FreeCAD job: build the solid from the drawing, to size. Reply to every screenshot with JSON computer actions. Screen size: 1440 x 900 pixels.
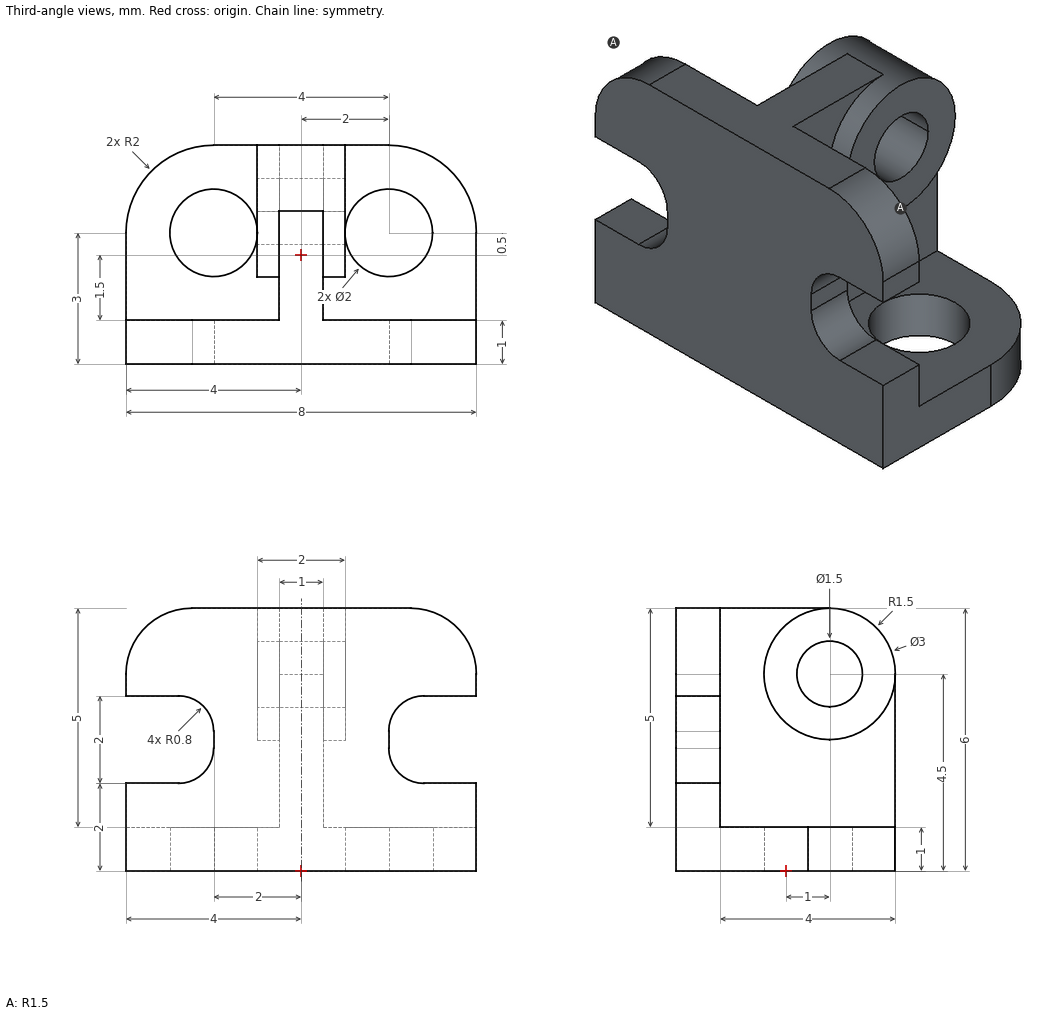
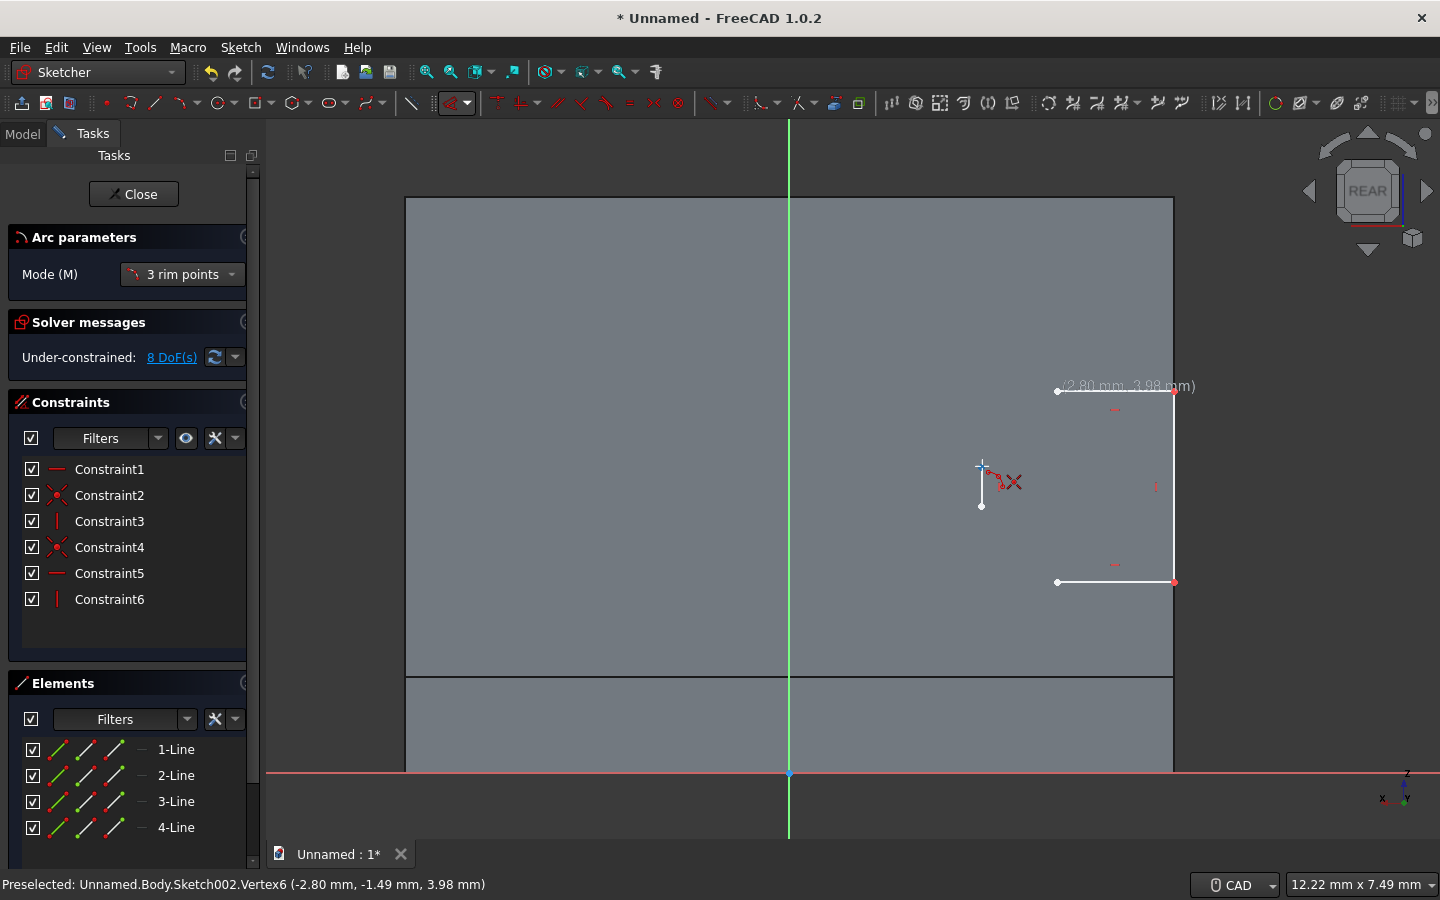
{"action": "left_click", "coordinate": [982, 467]}
{"action": "left_click", "coordinate": [1004, 412]}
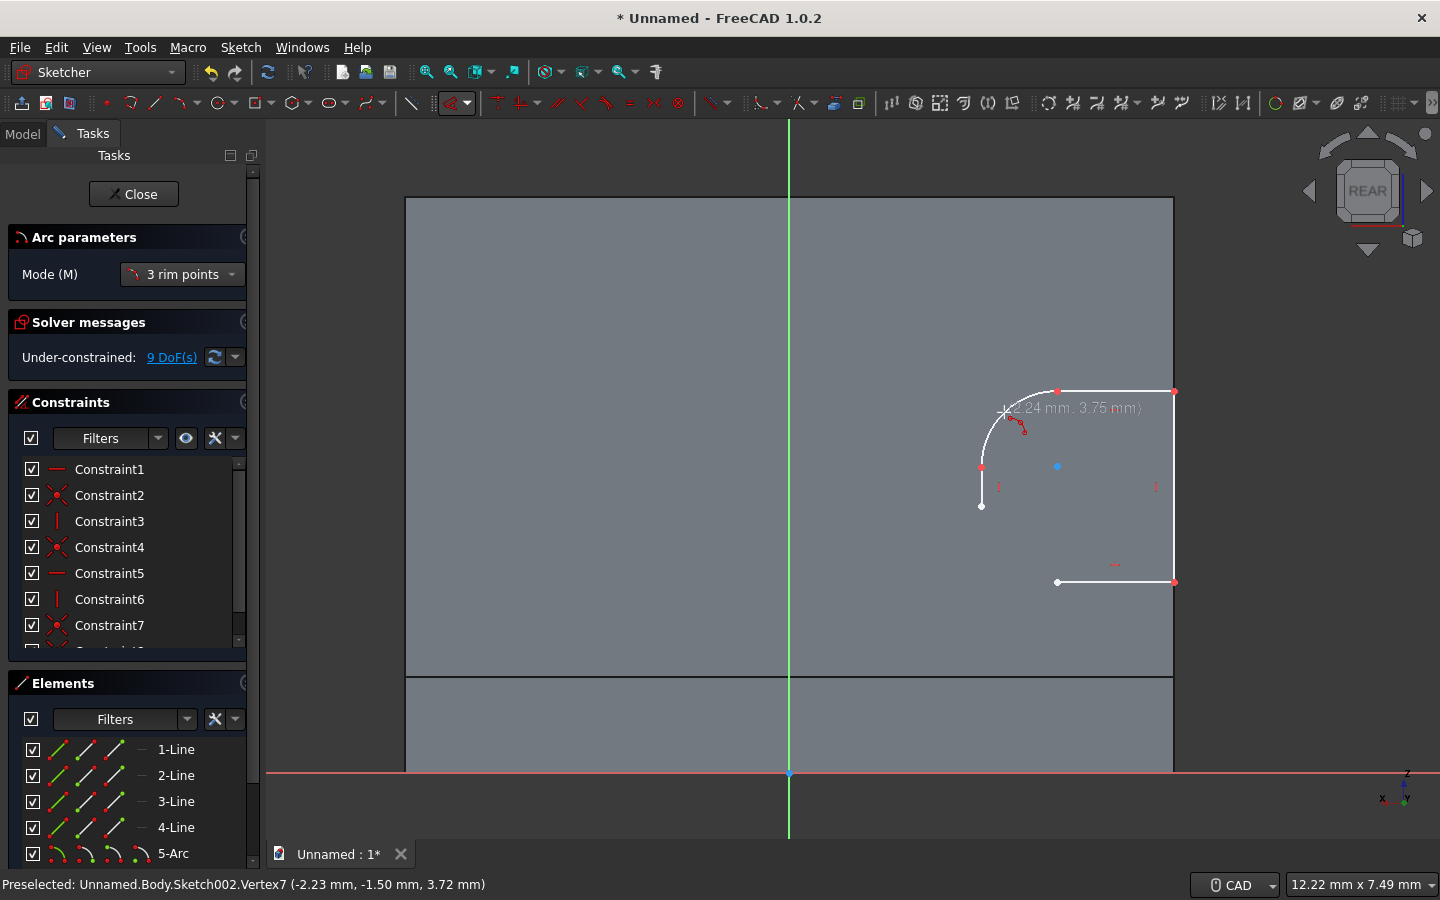
{"action": "left_click", "coordinate": [982, 506]}
{"action": "left_click", "coordinate": [1058, 582]}
{"action": "left_click", "coordinate": [1004, 559]}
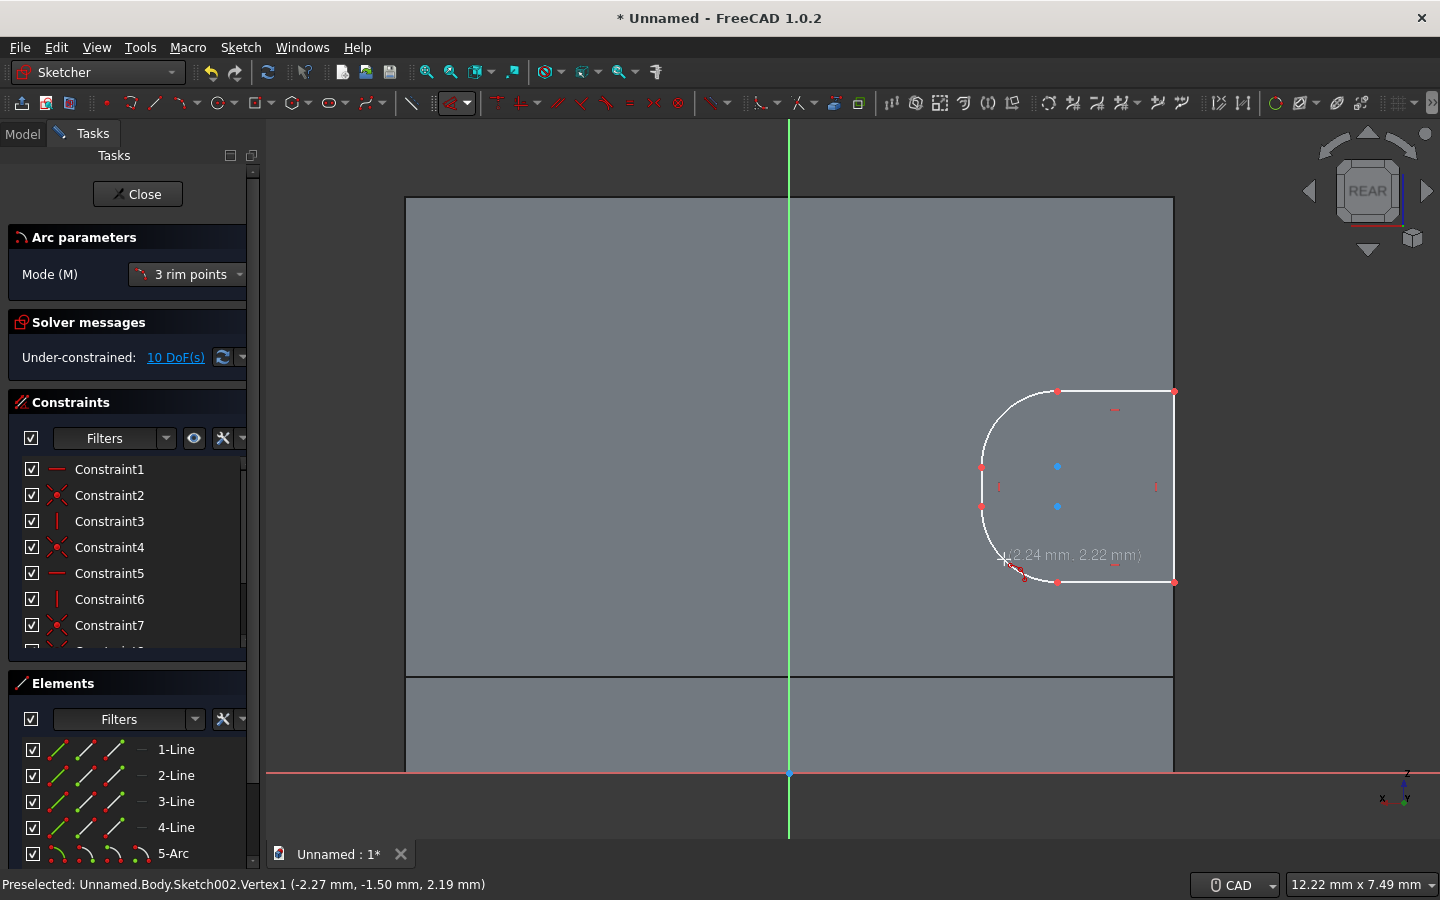
{"action": "left_click", "coordinate": [156, 104]}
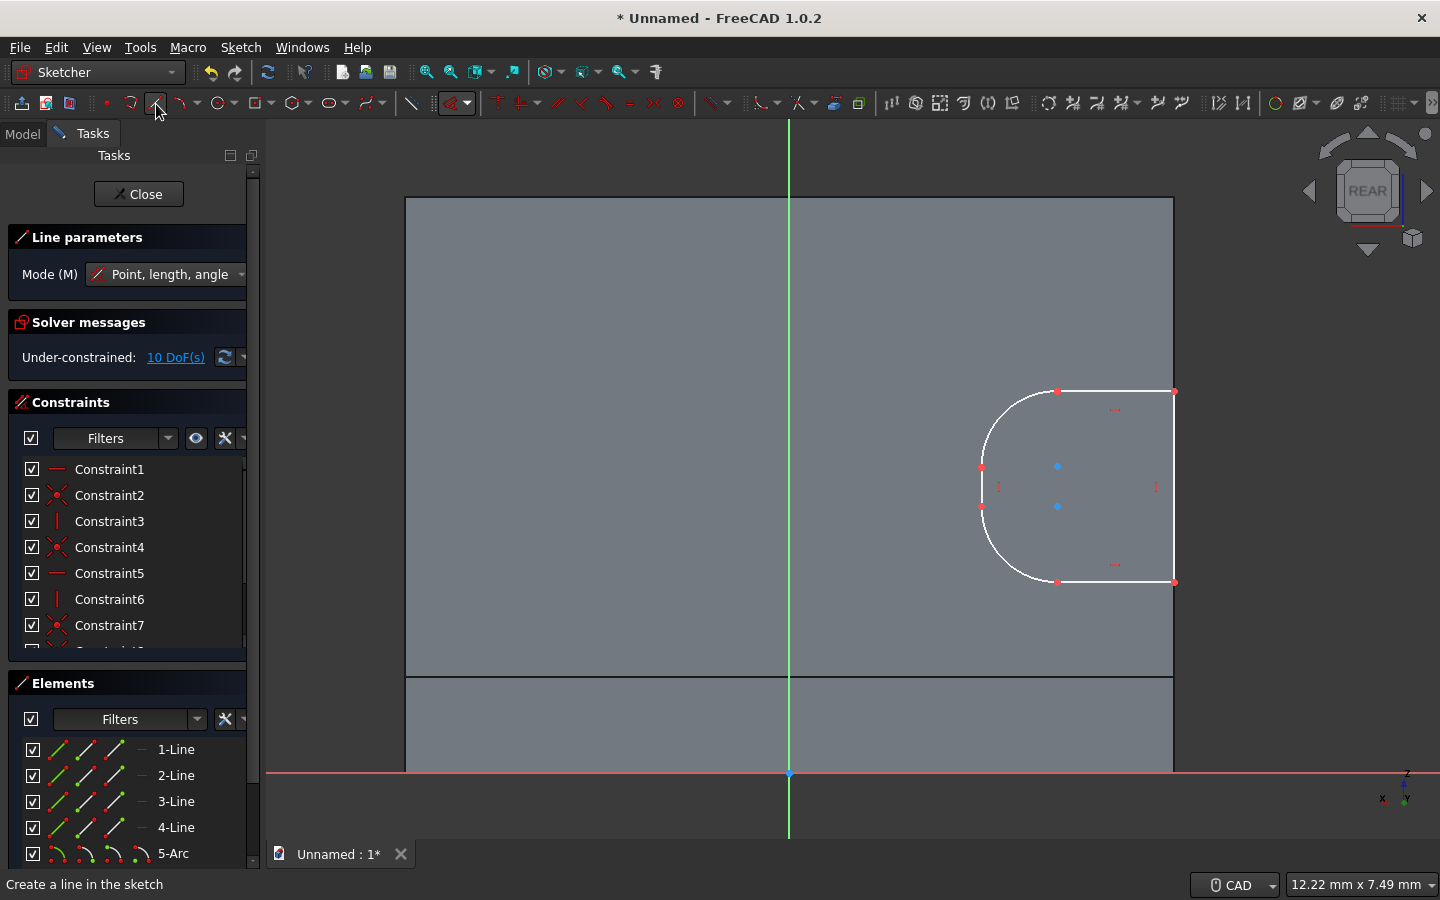
{"action": "left_click", "coordinate": [597, 504]}
{"action": "left_click", "coordinate": [597, 466]}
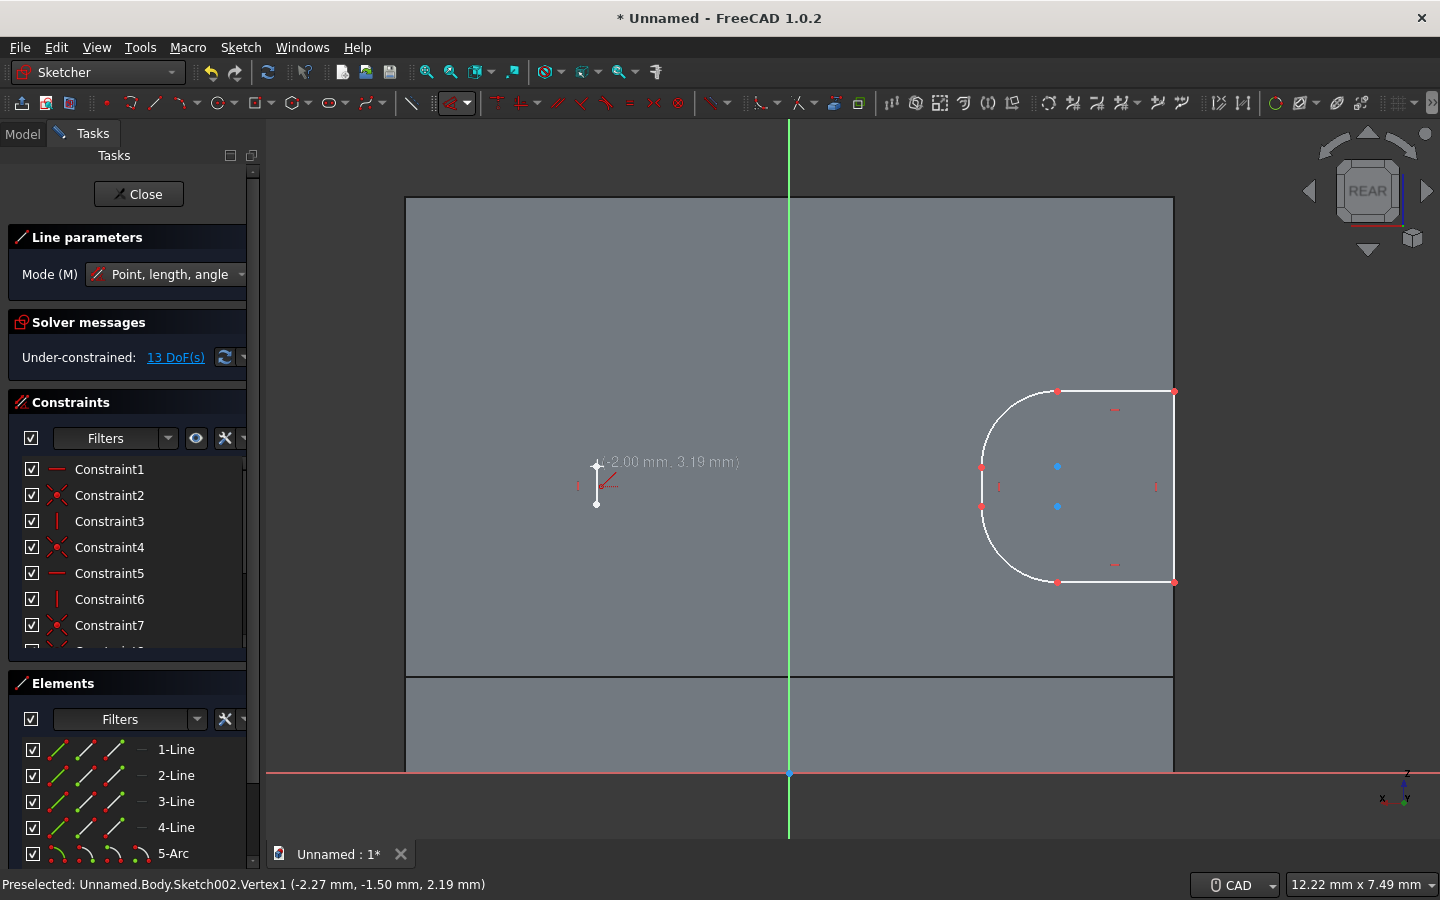
{"action": "left_click", "coordinate": [132, 104]}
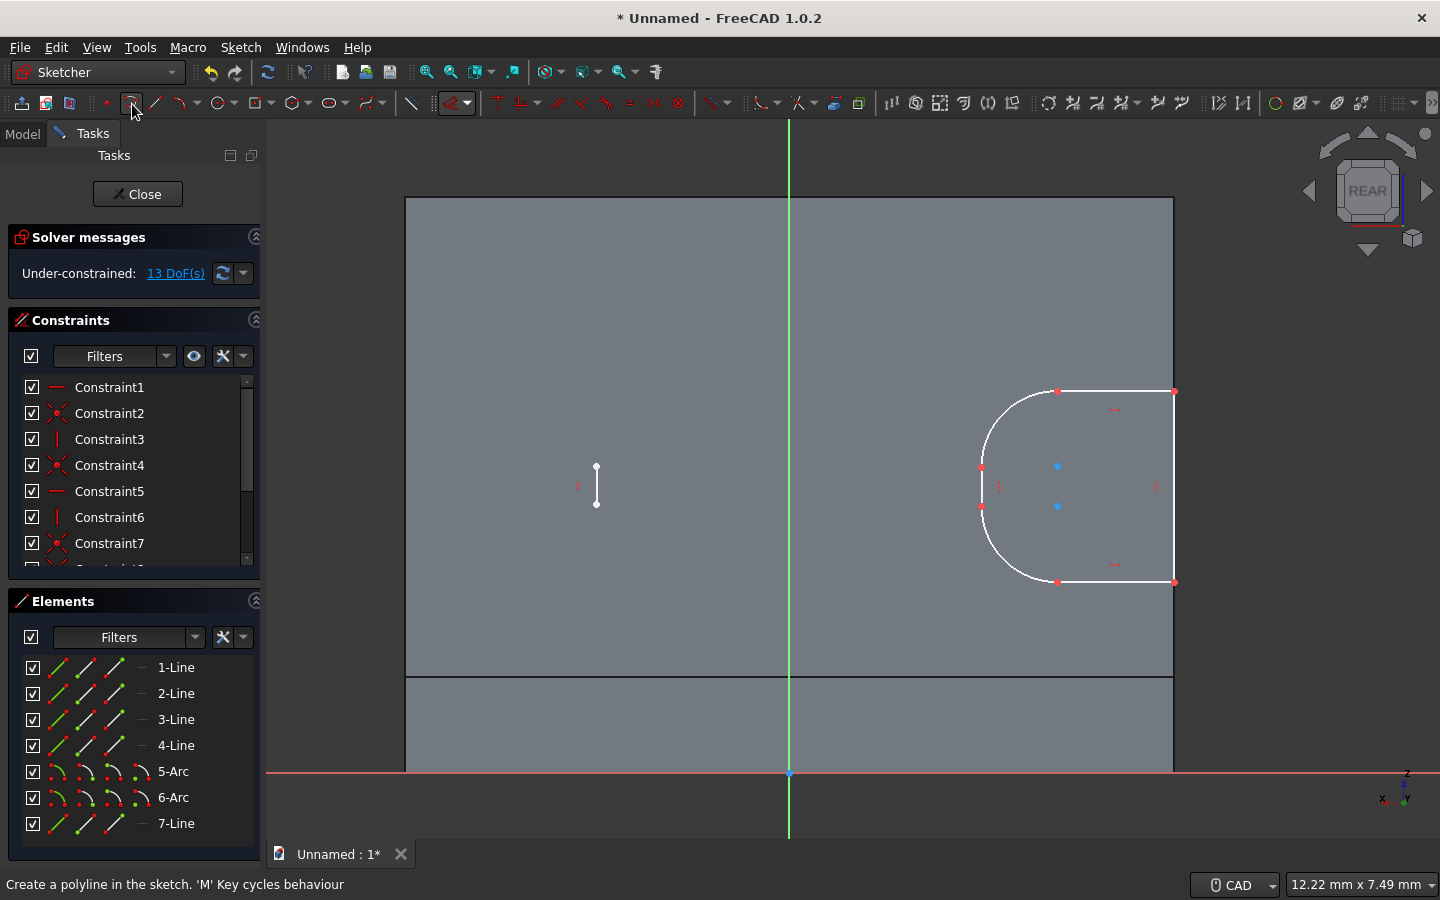
{"action": "left_click", "coordinate": [520, 389]}
{"action": "left_click", "coordinate": [405, 389]}
{"action": "left_click", "coordinate": [405, 581]}
{"action": "left_click", "coordinate": [520, 581]}
{"action": "right_click", "coordinate": [520, 581]}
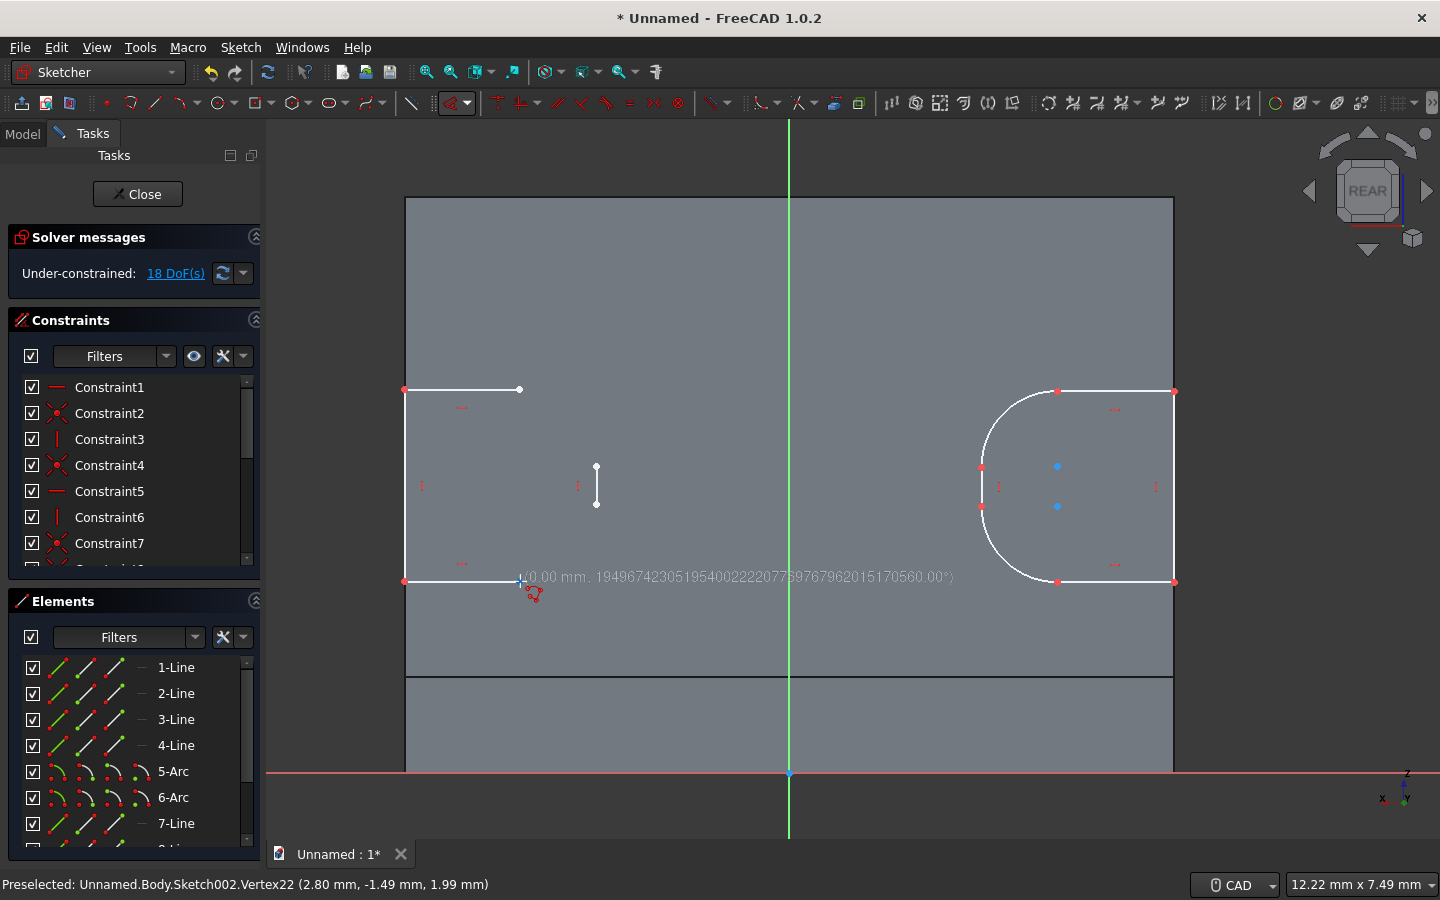
{"action": "left_click", "coordinate": [180, 104]}